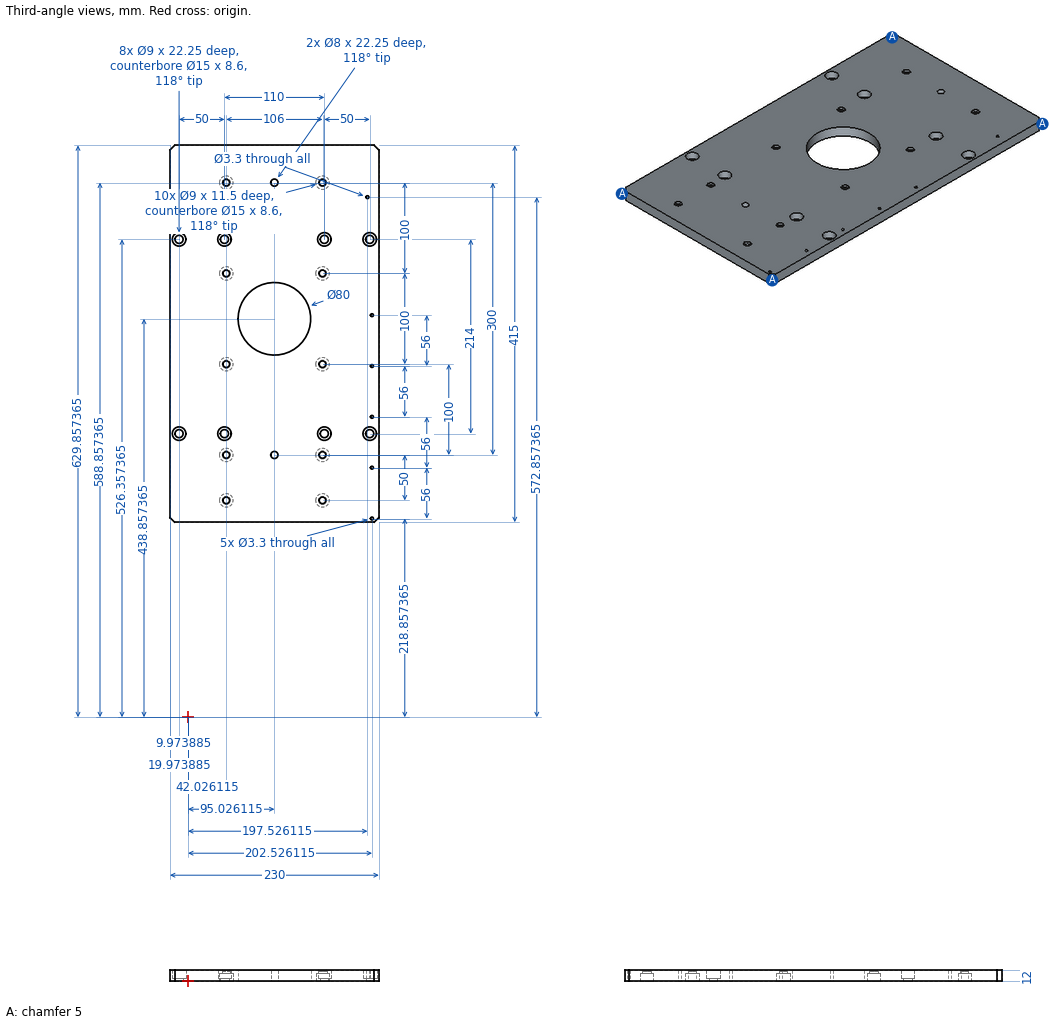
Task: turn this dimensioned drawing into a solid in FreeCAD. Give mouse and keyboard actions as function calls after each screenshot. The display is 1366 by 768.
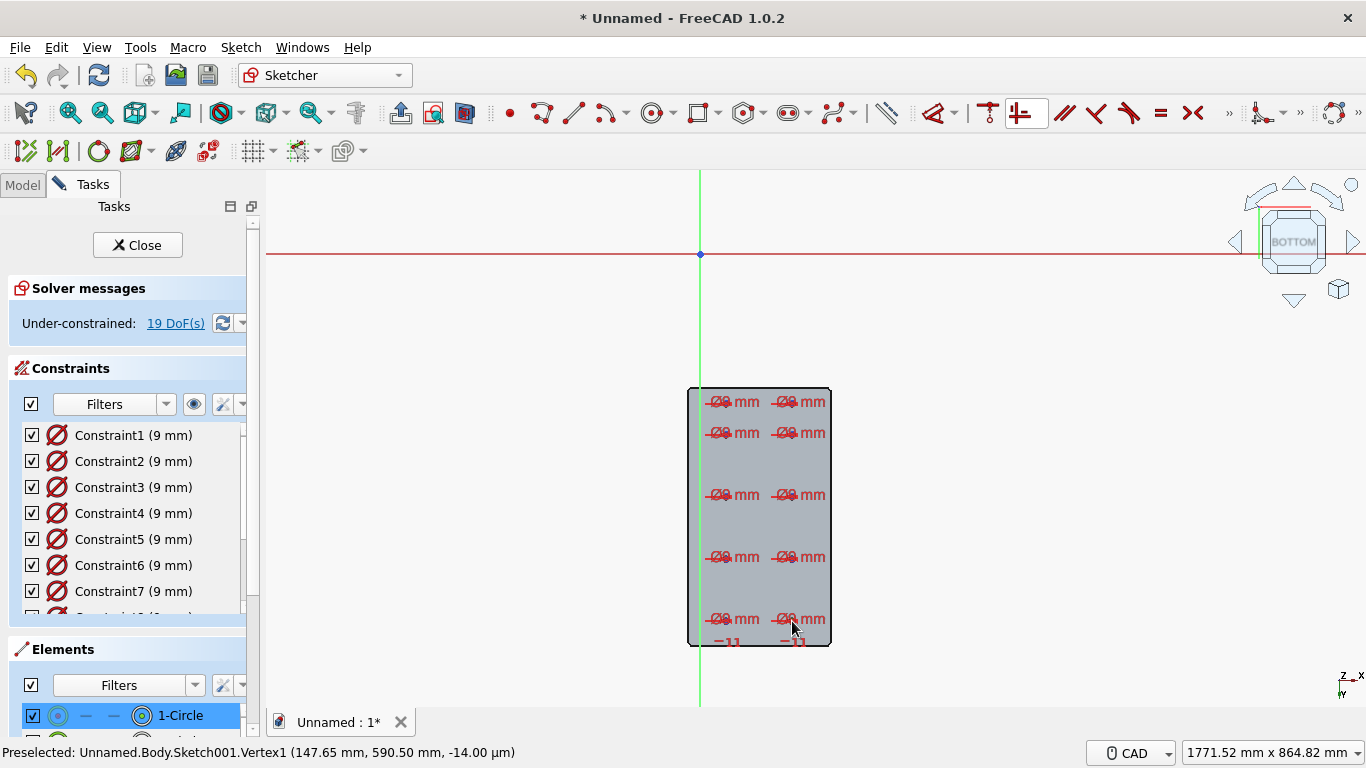
click(792, 559)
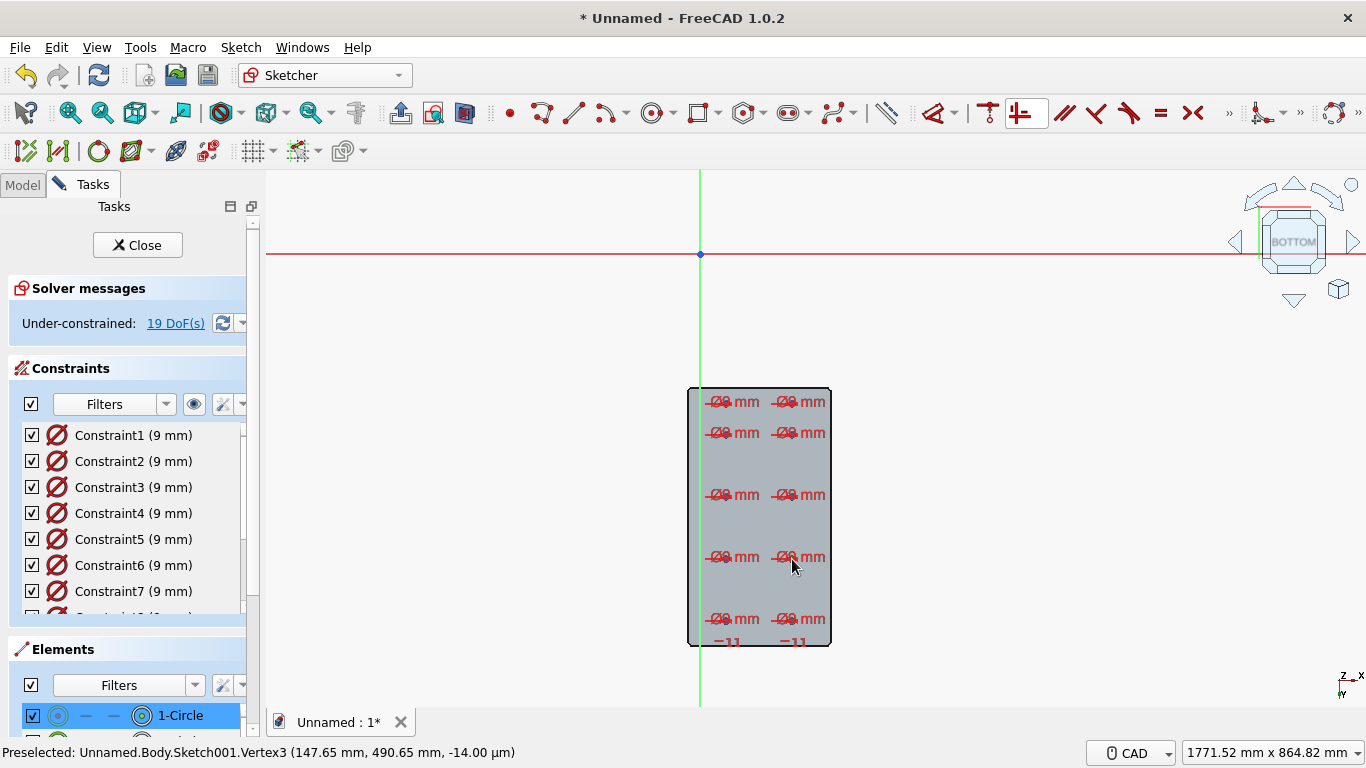
key(v)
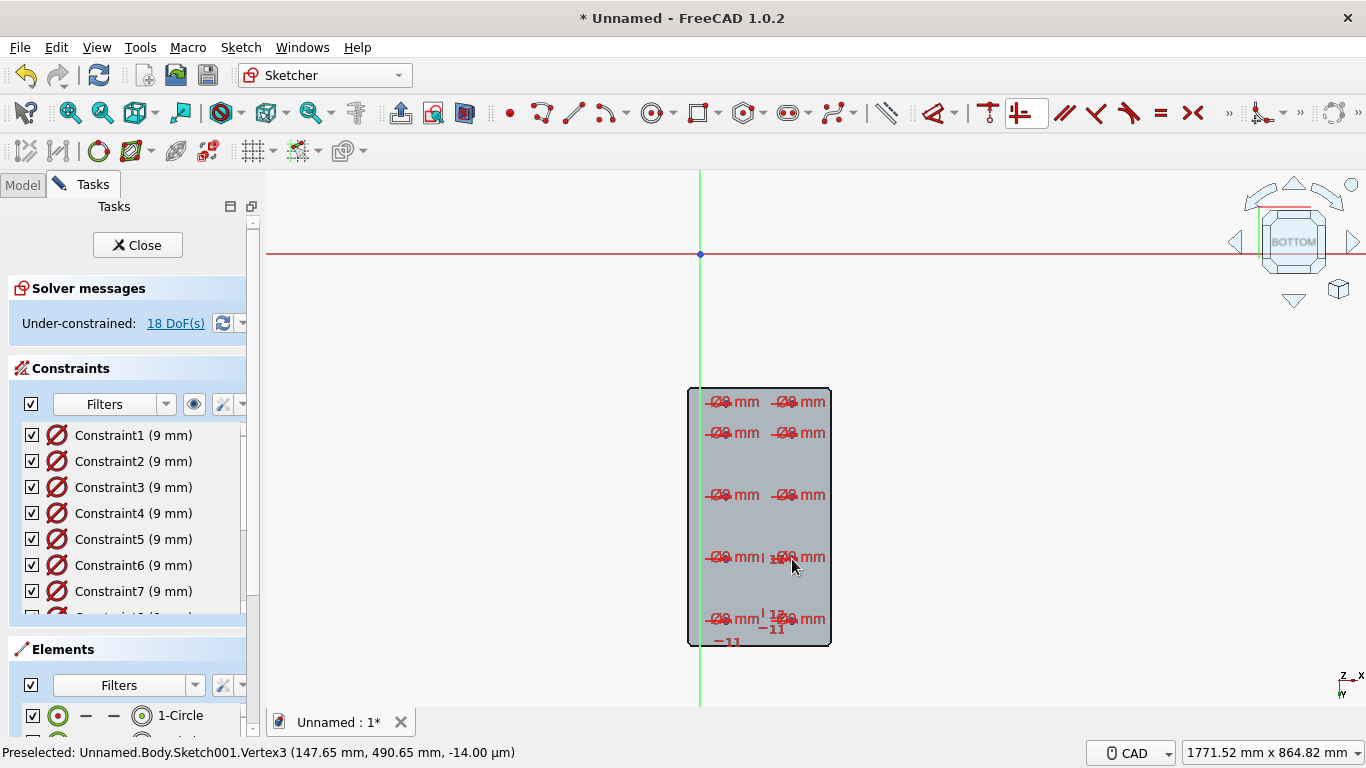
click(726, 621)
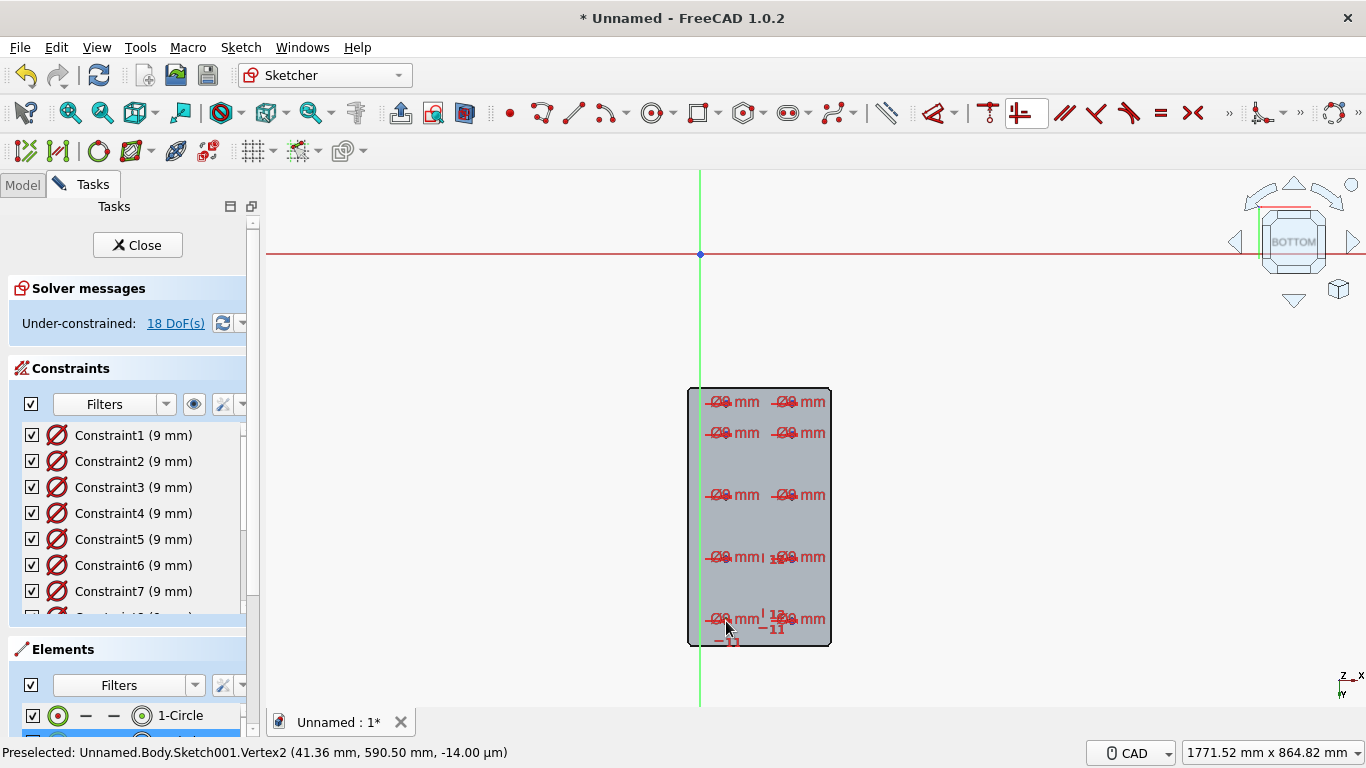
click(726, 559)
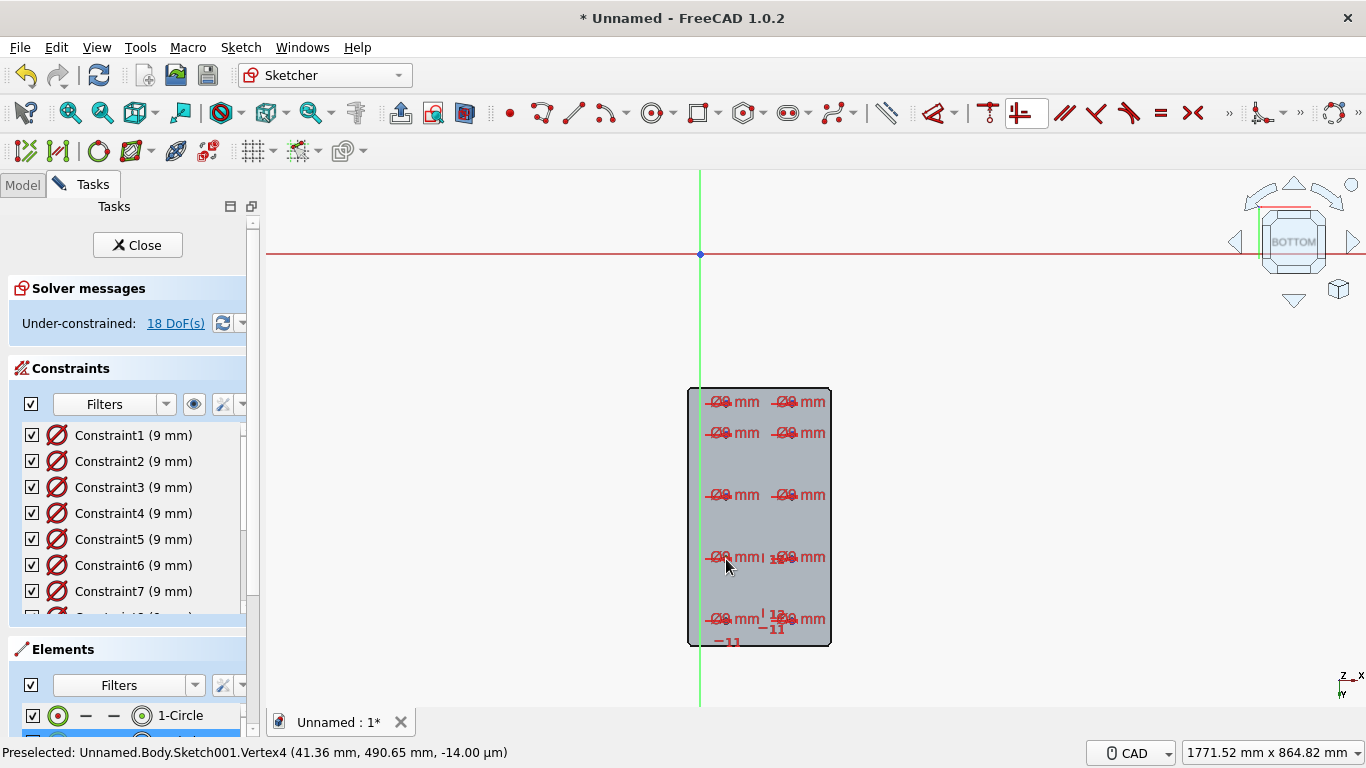
click(1042, 114)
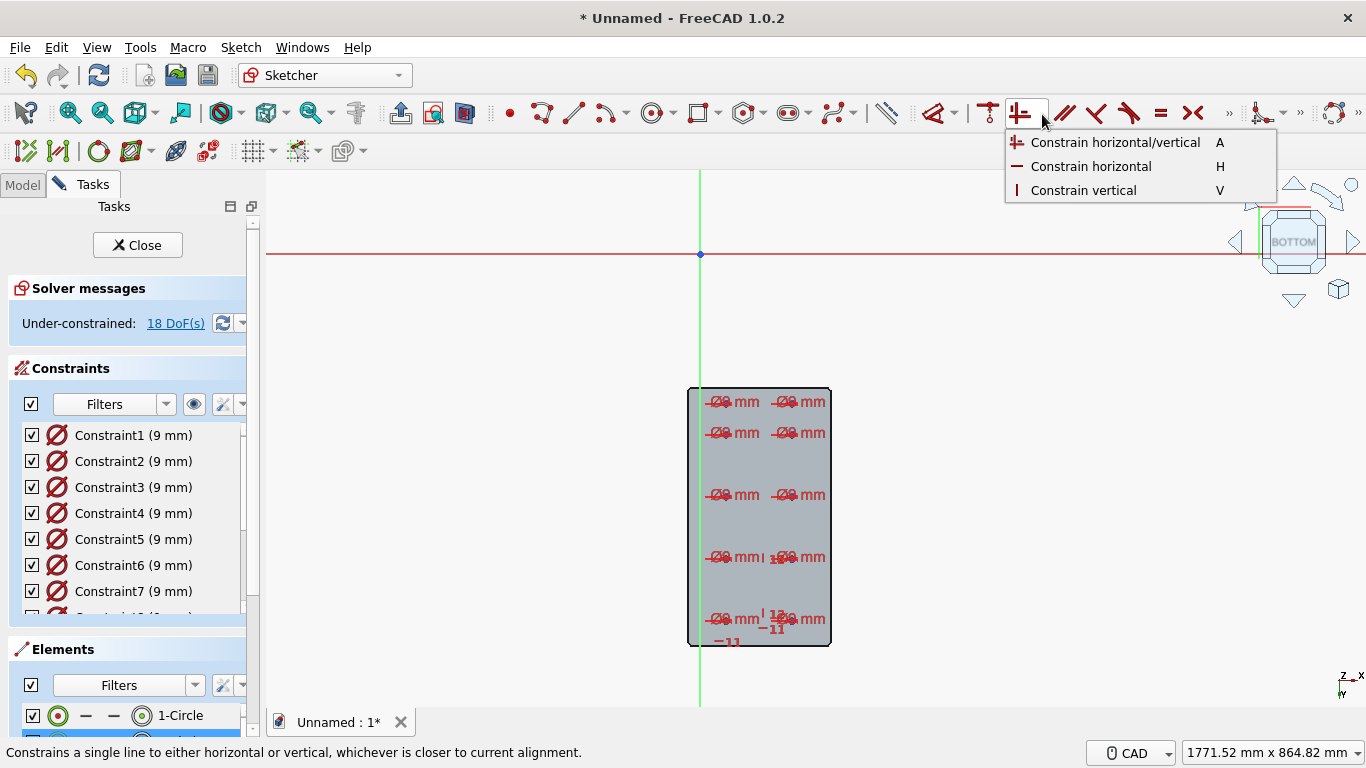
click(1141, 190)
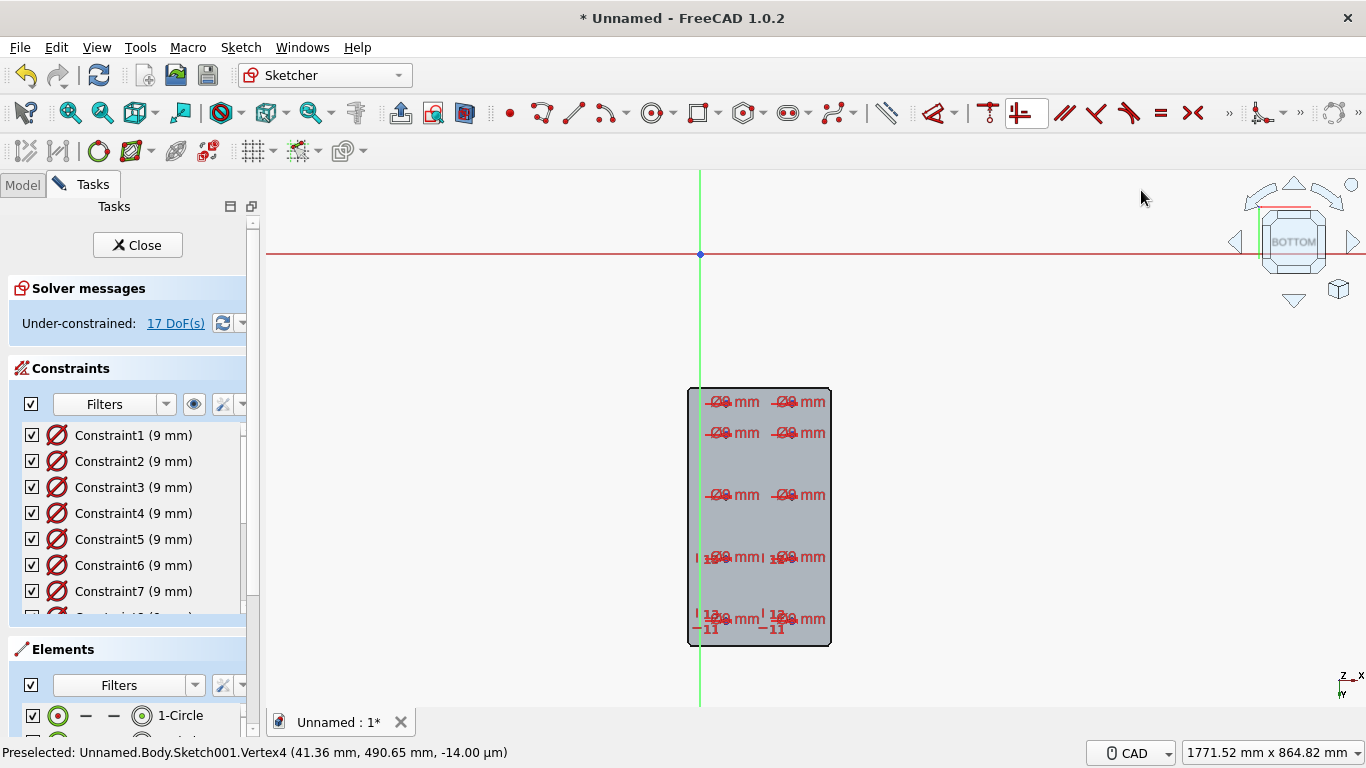
click(792, 559)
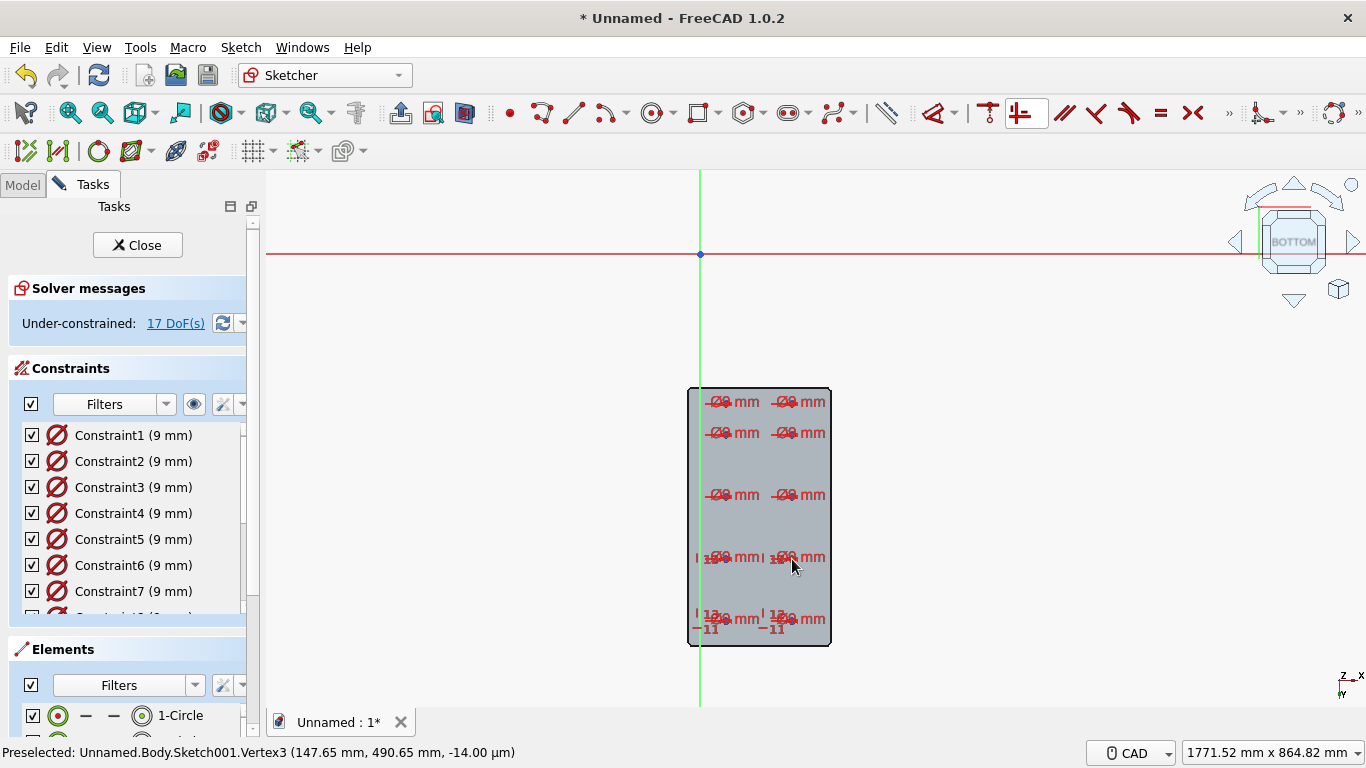
click(726, 559)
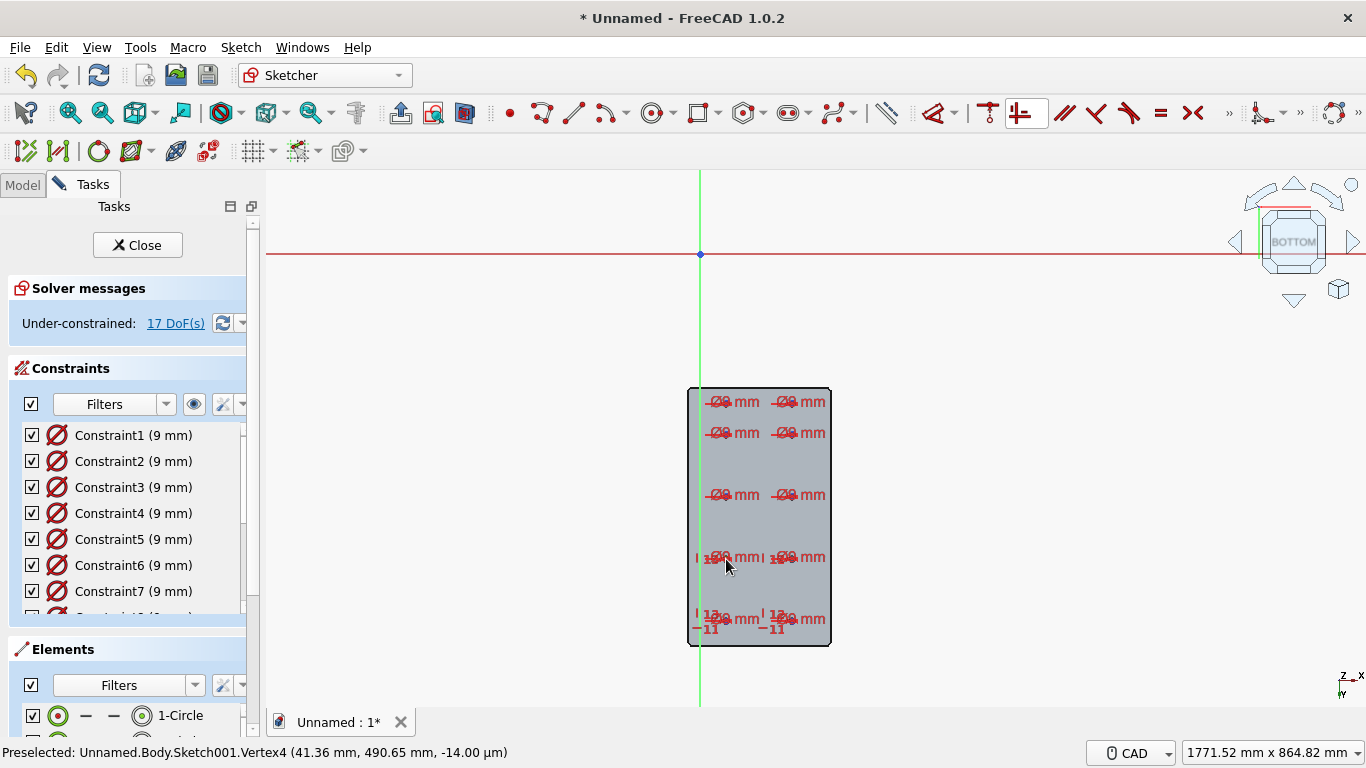
key(h)